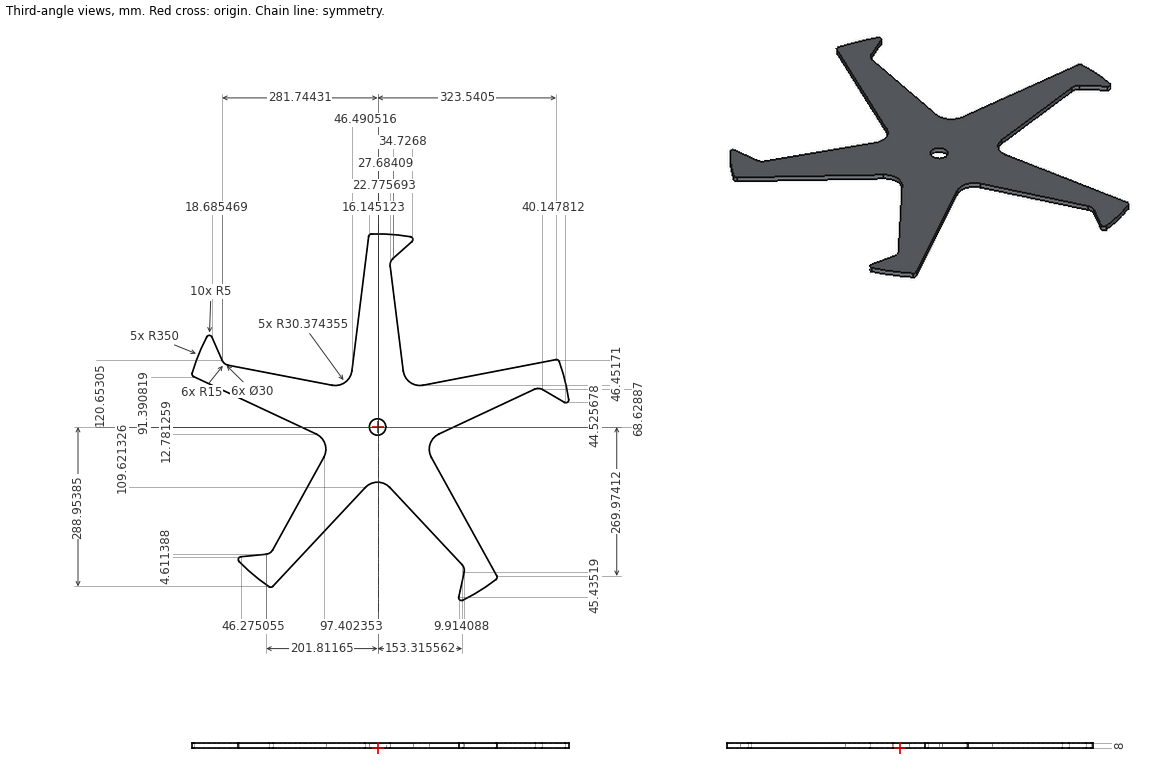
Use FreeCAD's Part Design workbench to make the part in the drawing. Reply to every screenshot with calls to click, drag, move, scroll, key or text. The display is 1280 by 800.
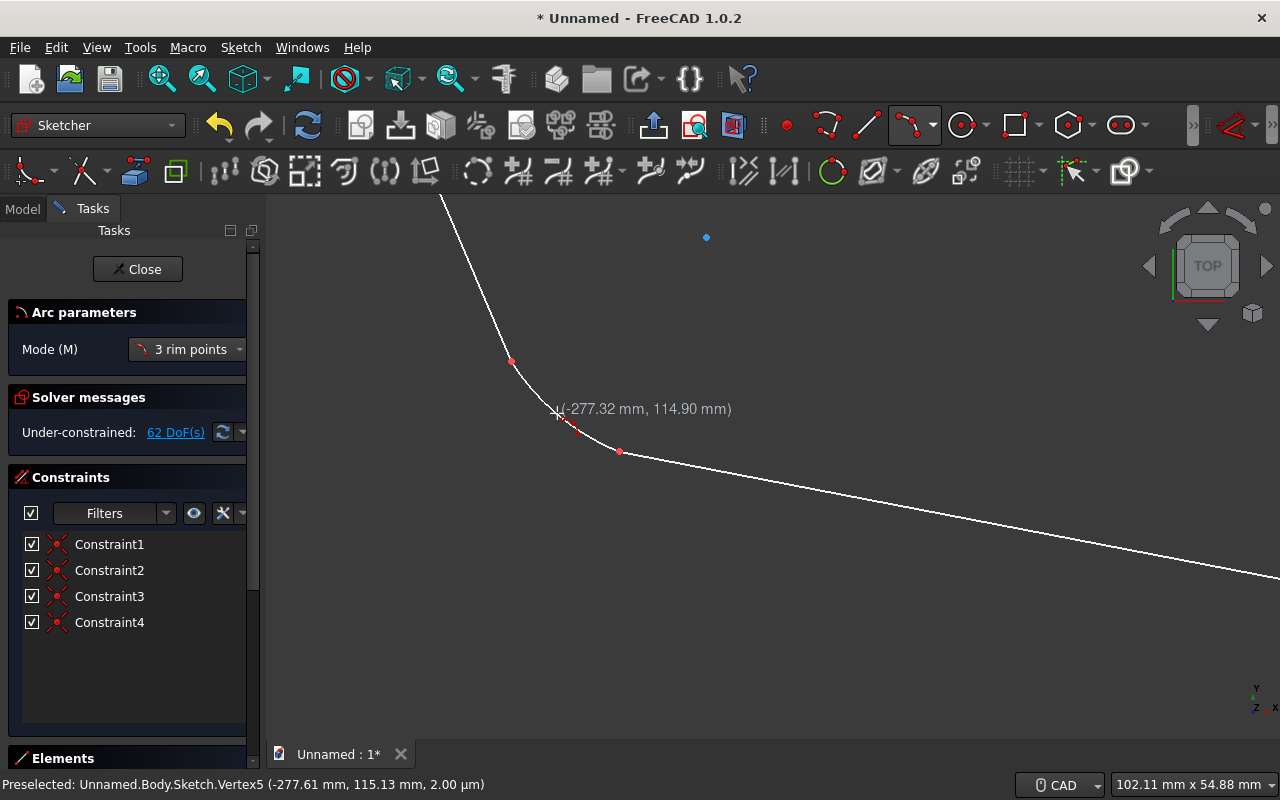
scroll(565, 419, down, 15)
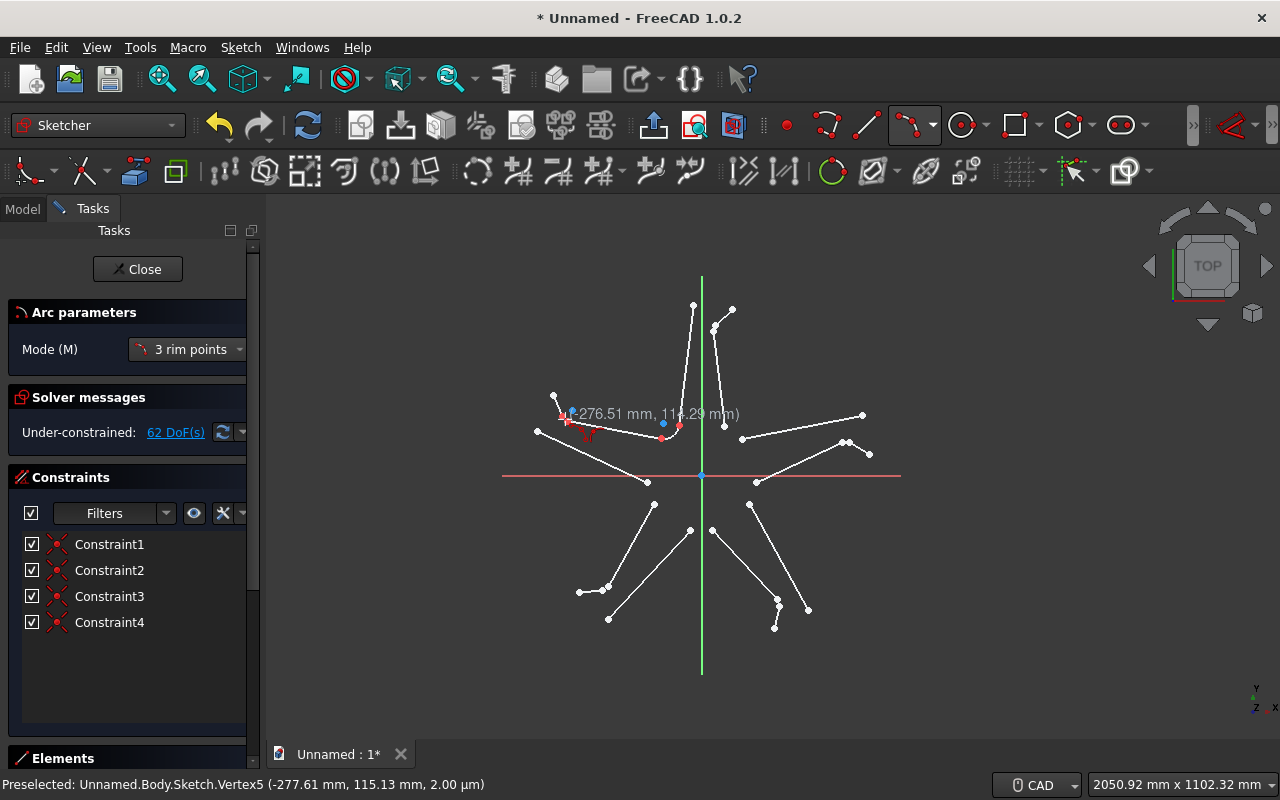
scroll(553, 395, up, 2)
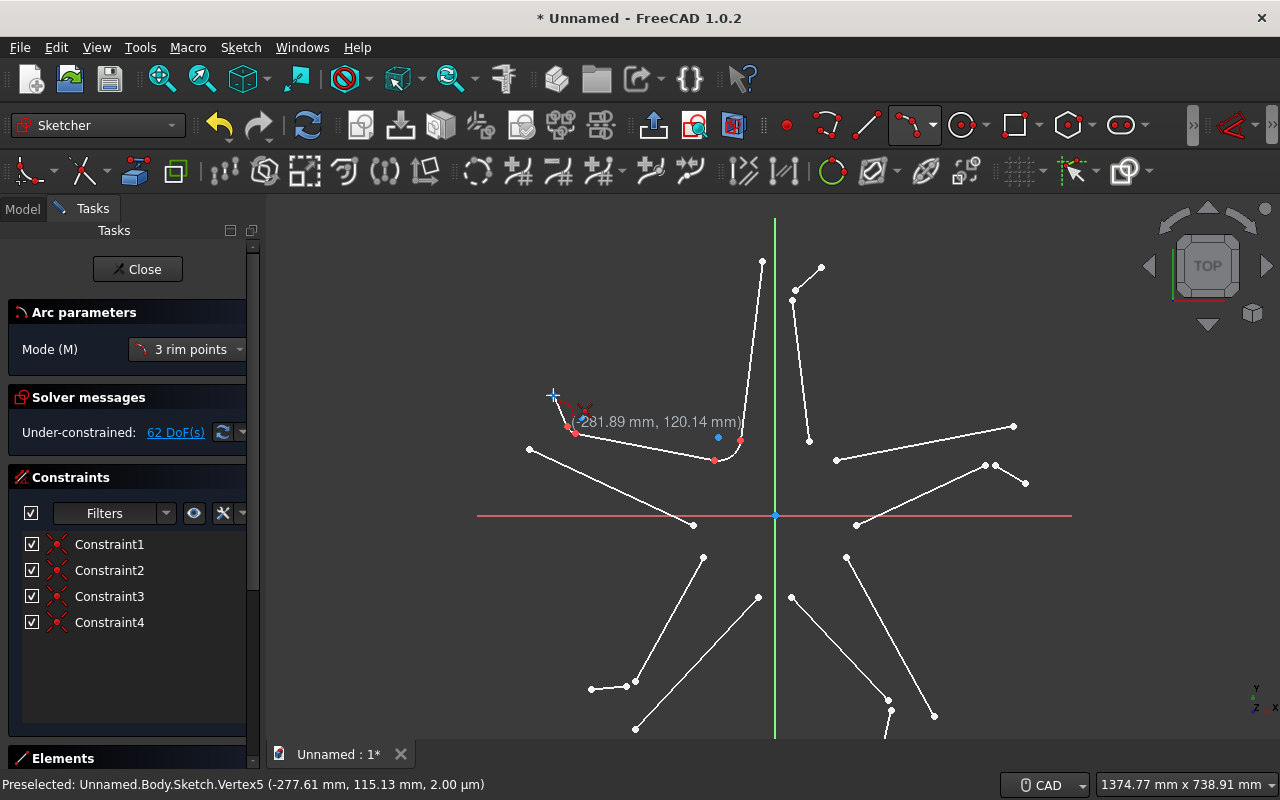
click(554, 396)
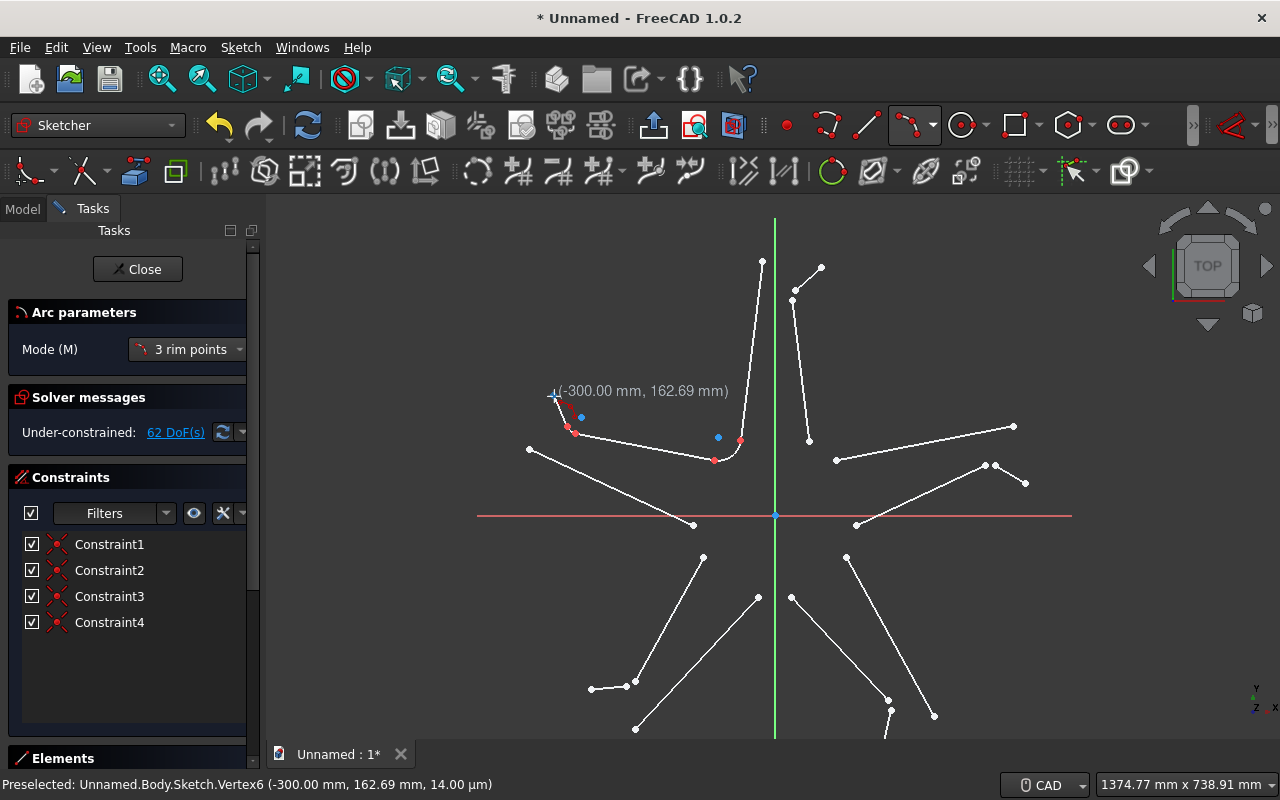
scroll(547, 395, up, 5)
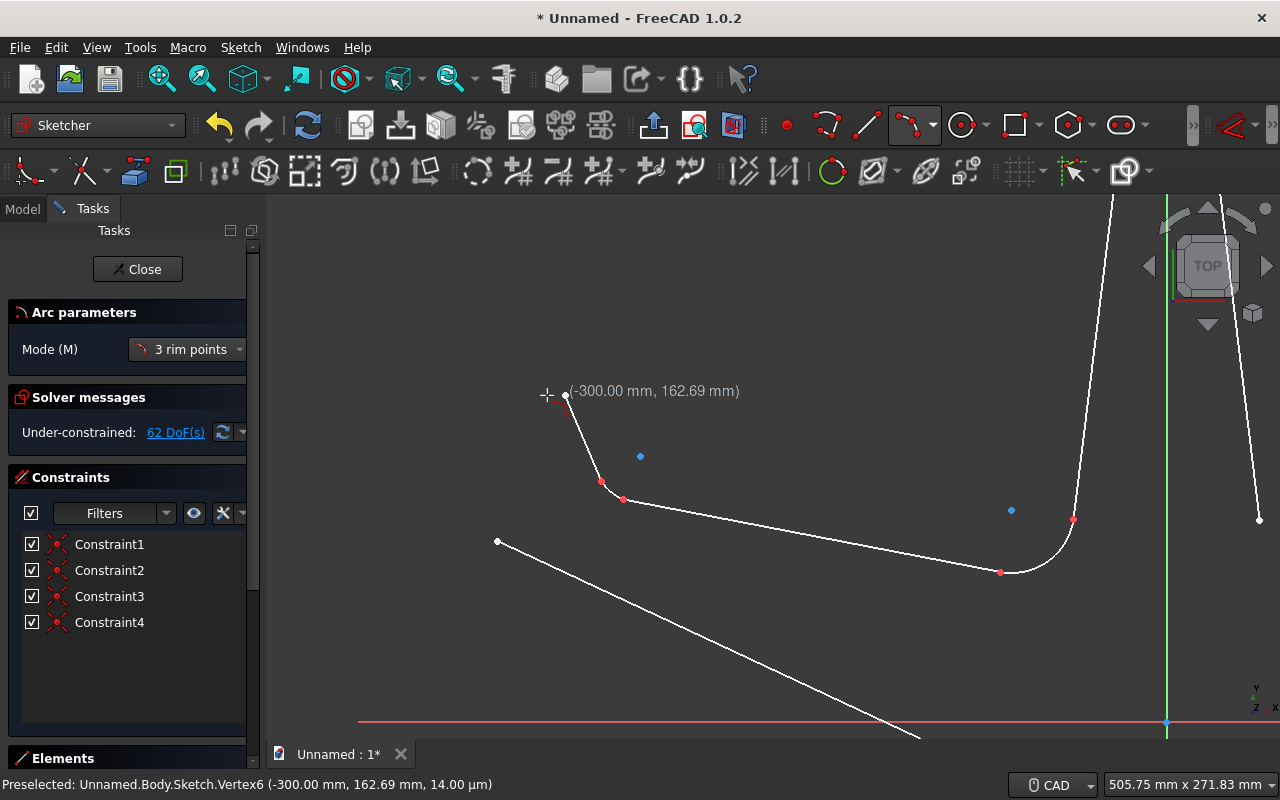
click(546, 394)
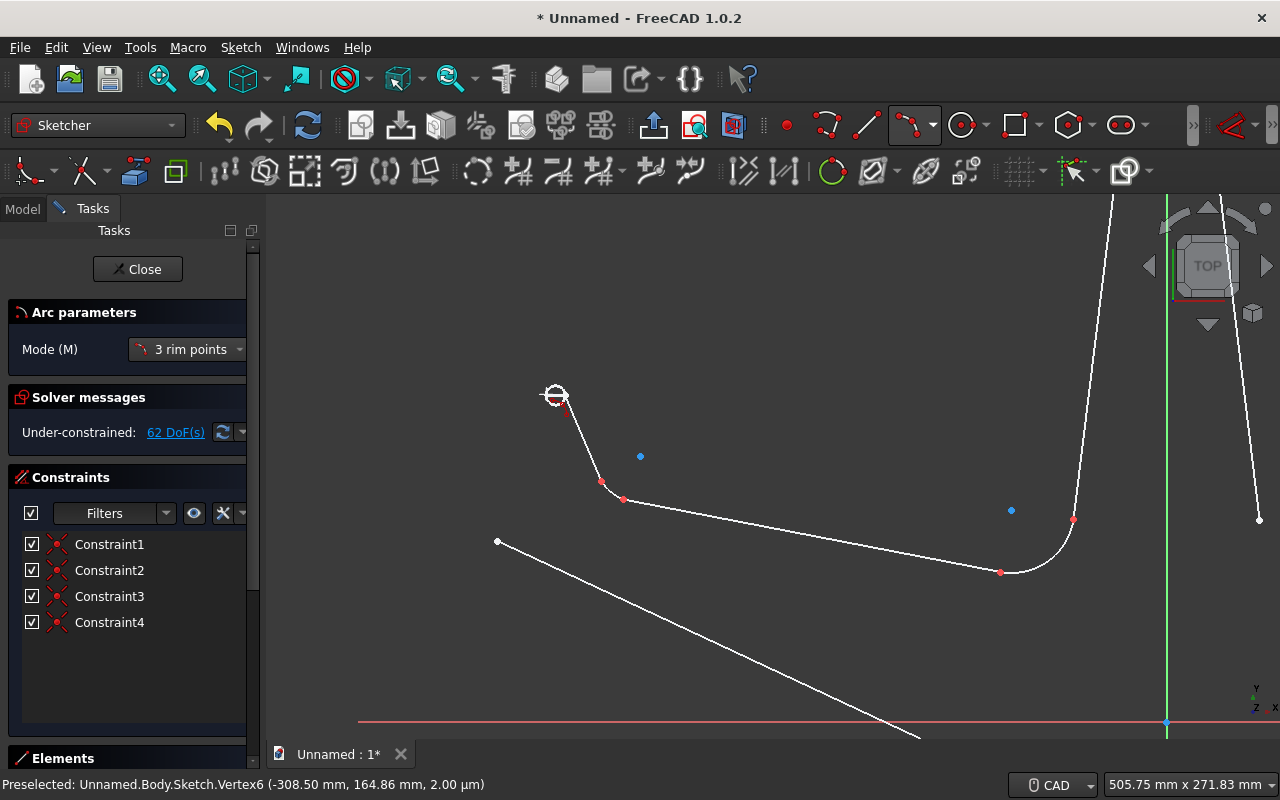
scroll(555, 389, up, 6)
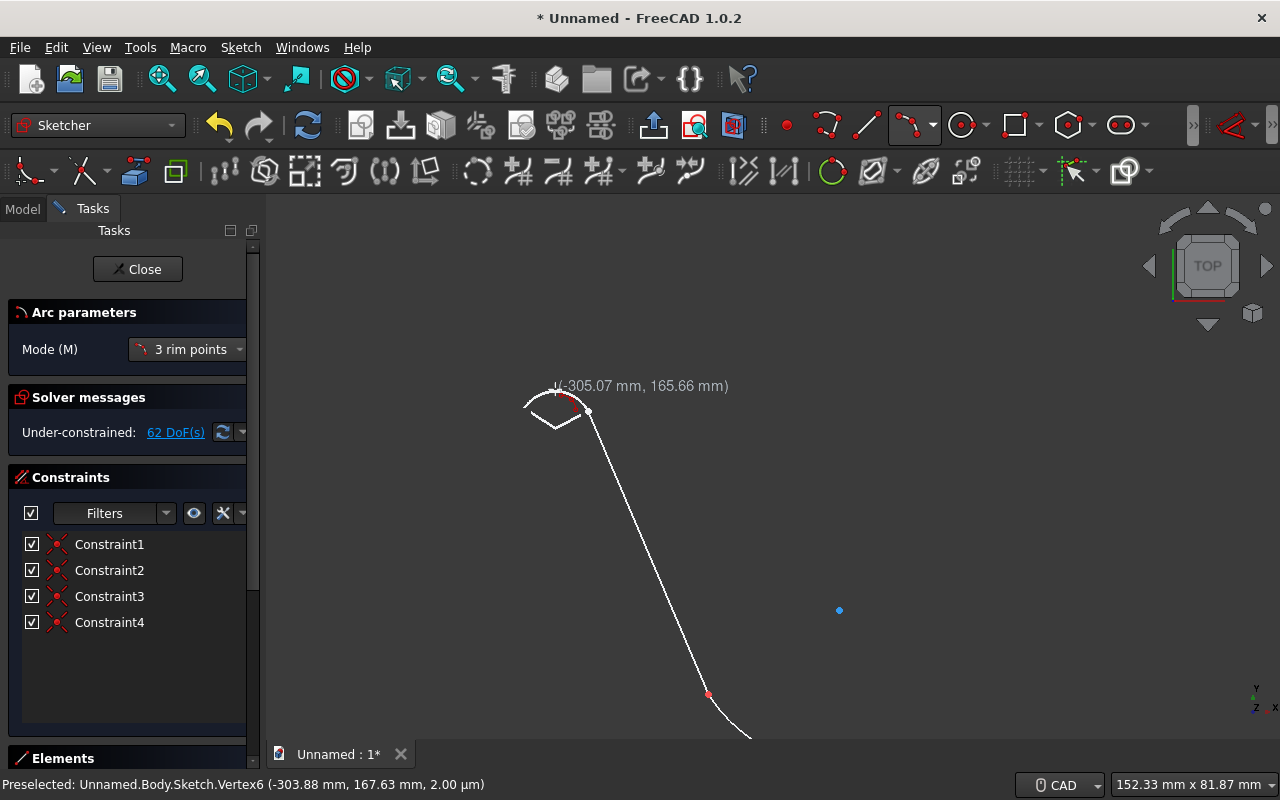
click(556, 388)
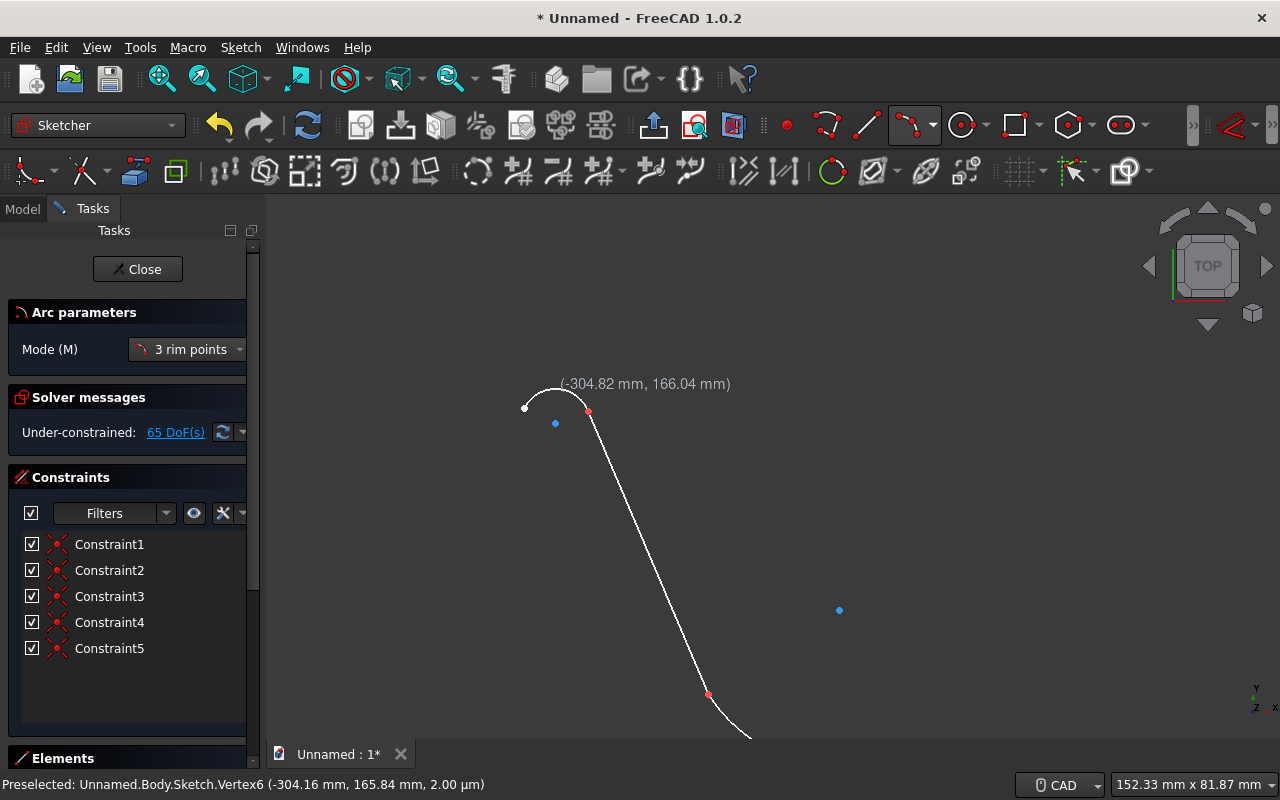
click(524, 408)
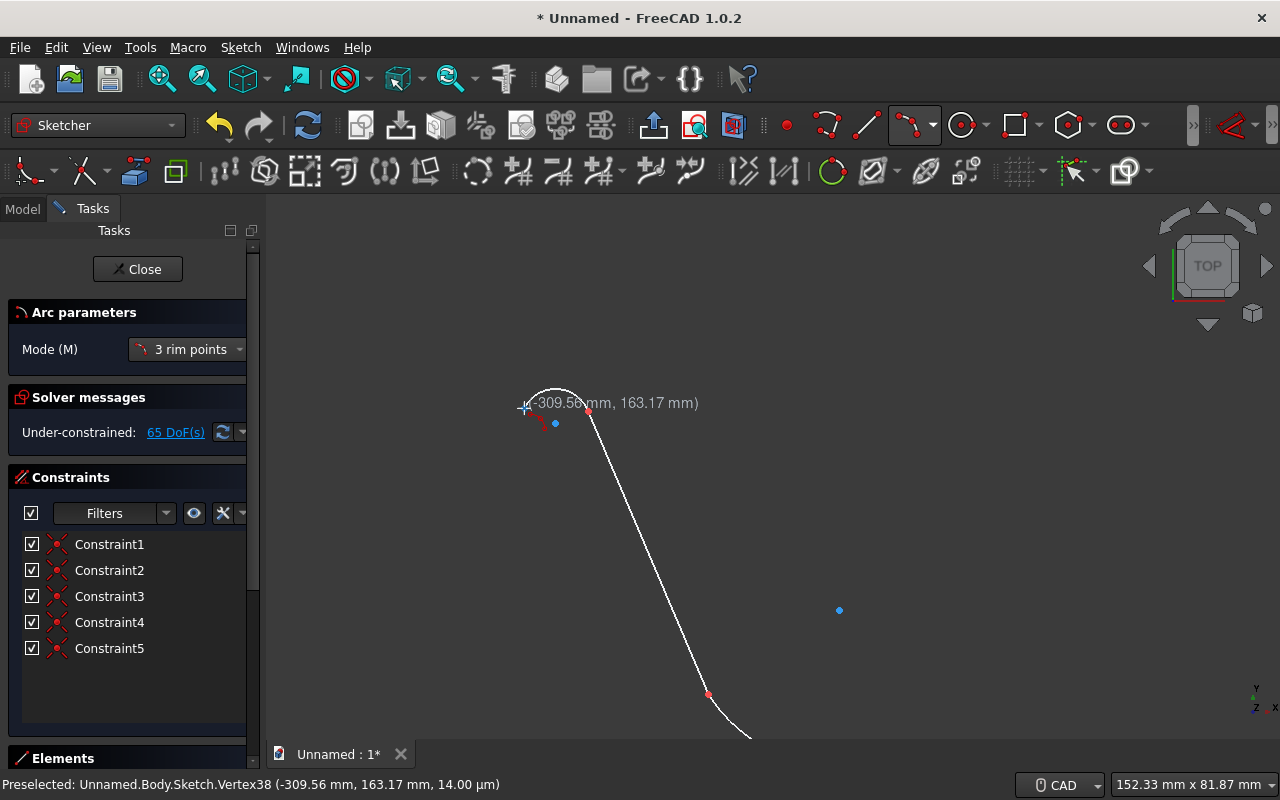
scroll(551, 394, down, 13)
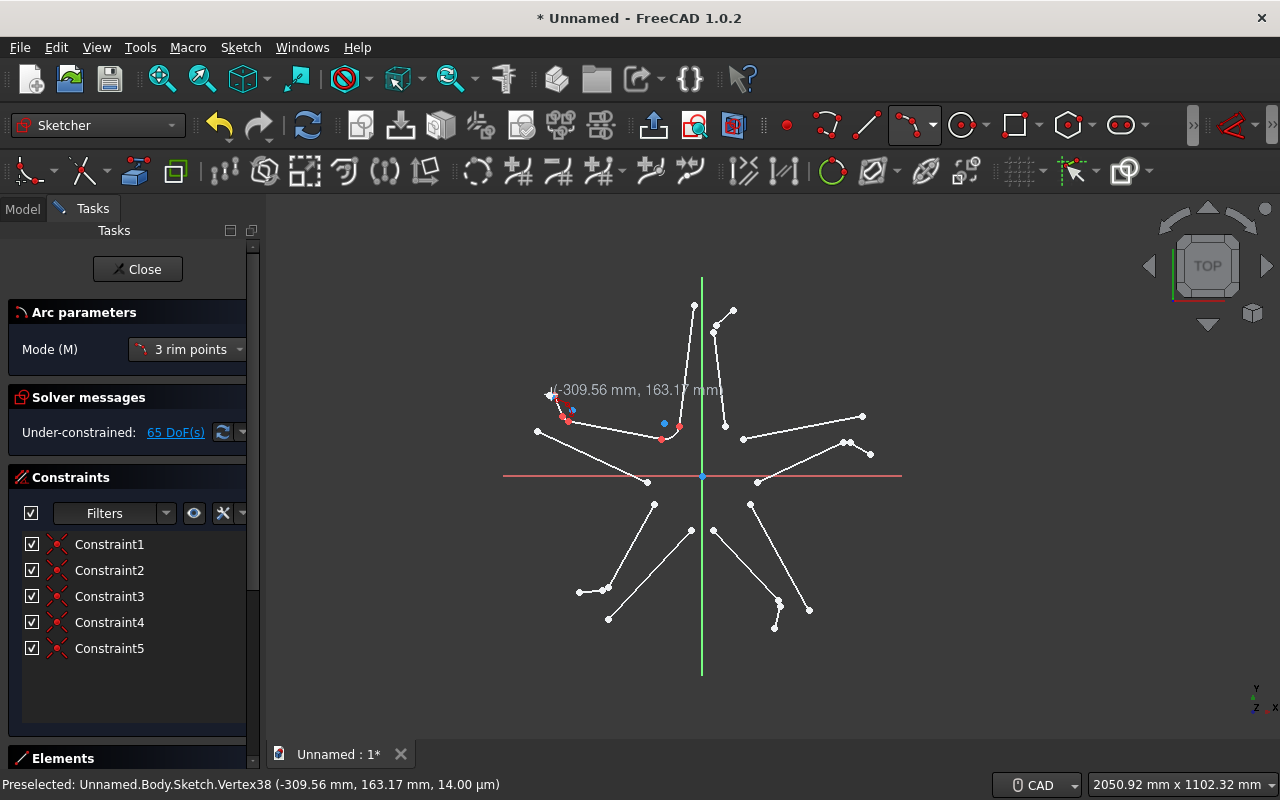
scroll(536, 428, up, 8)